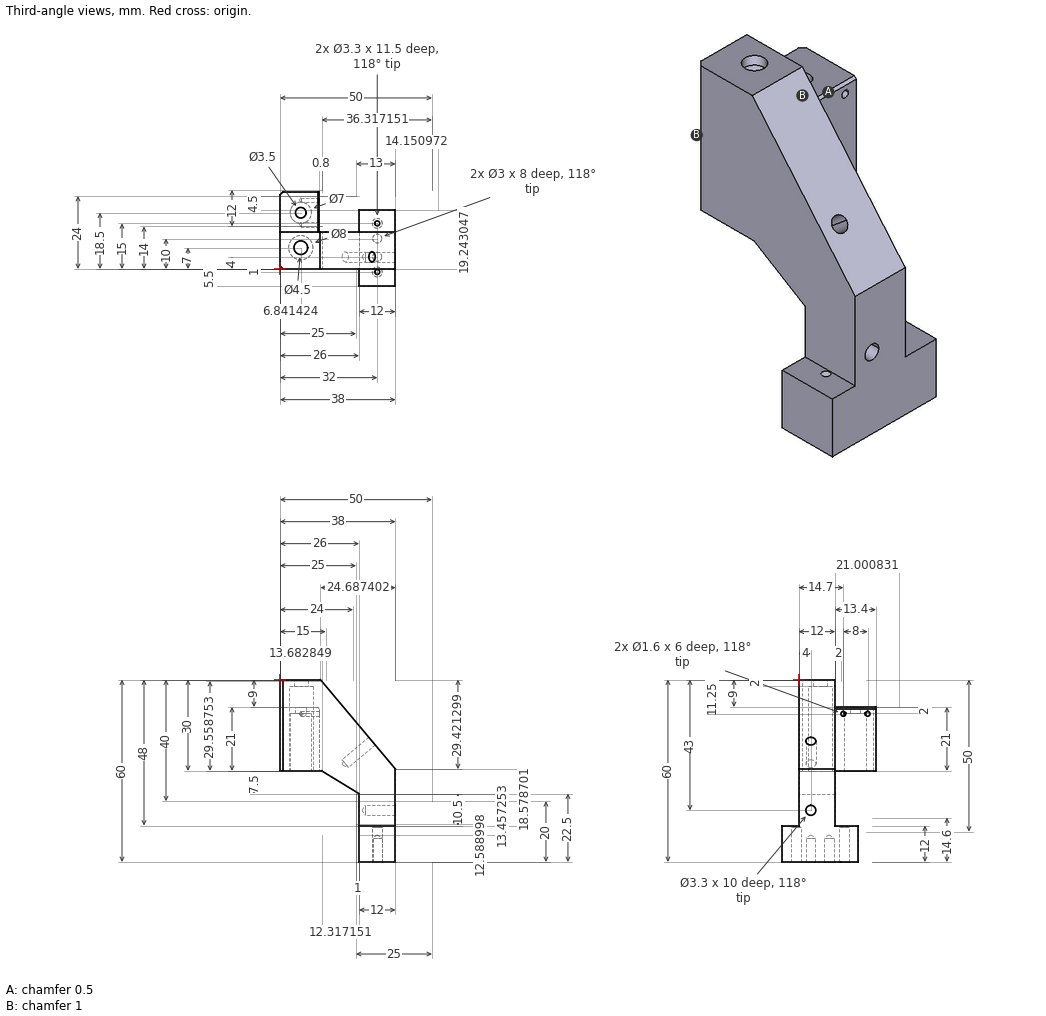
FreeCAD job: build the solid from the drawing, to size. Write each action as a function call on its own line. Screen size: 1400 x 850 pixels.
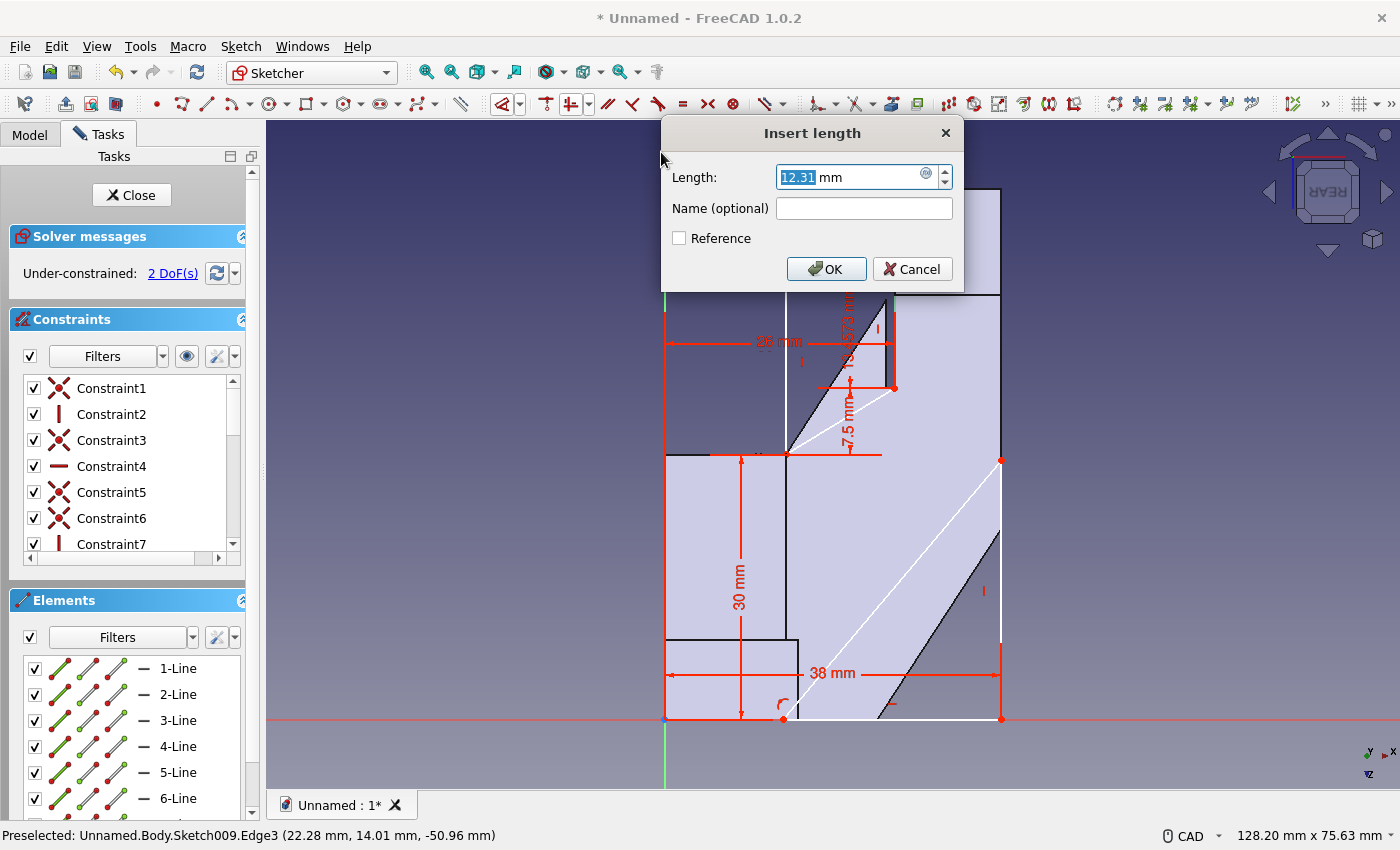
text(12.317151)
key(Return)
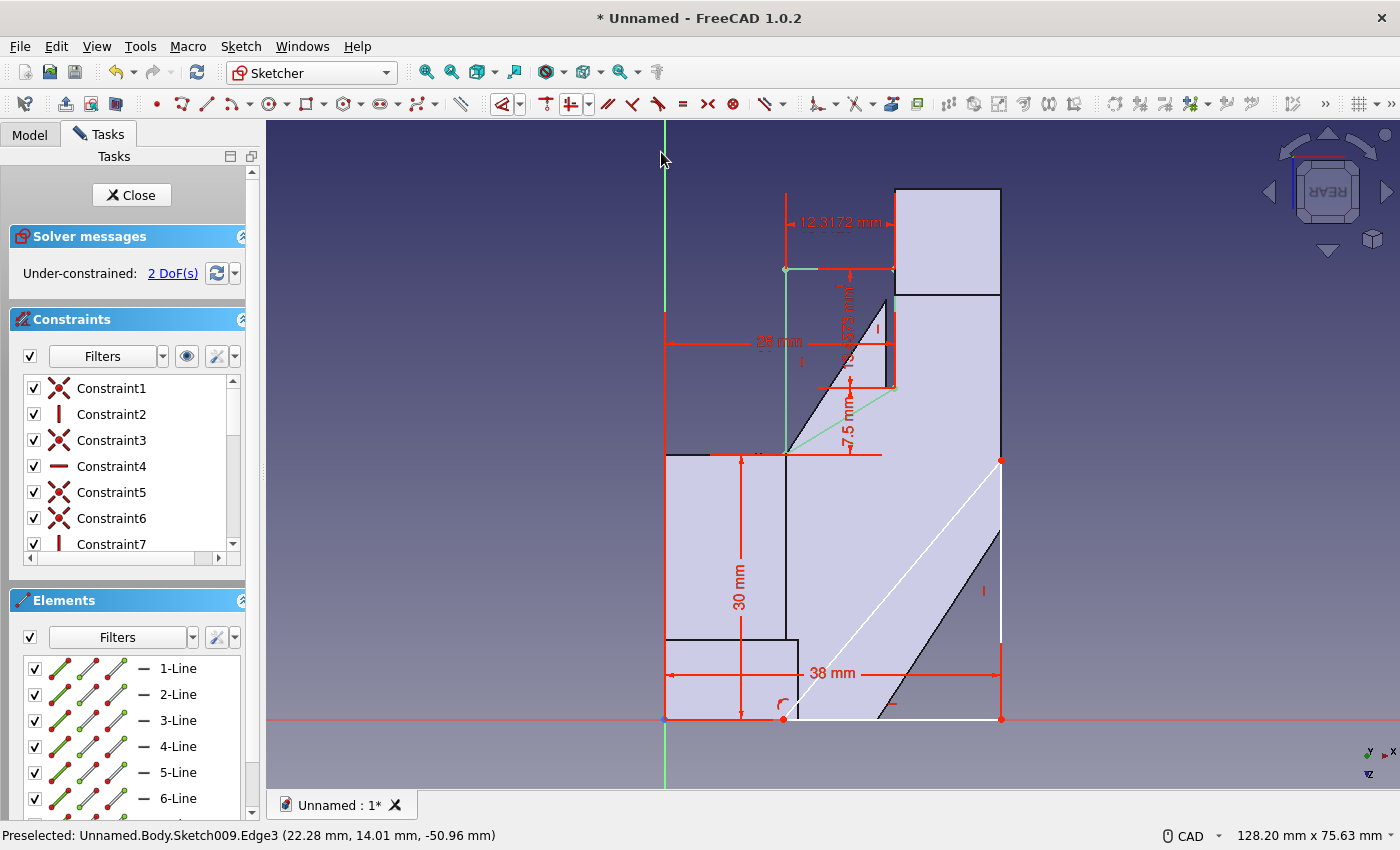
click(848, 720)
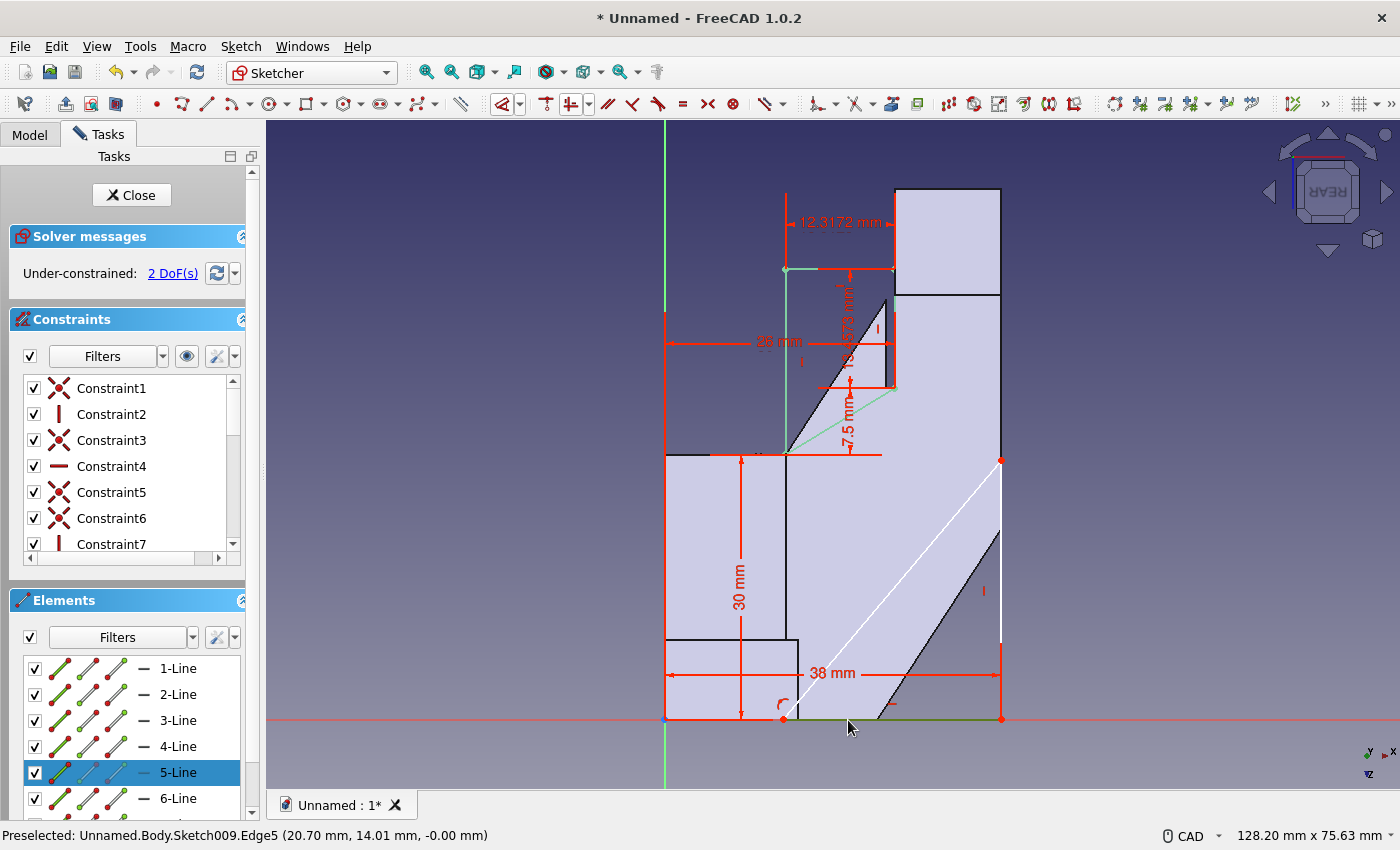
key(l)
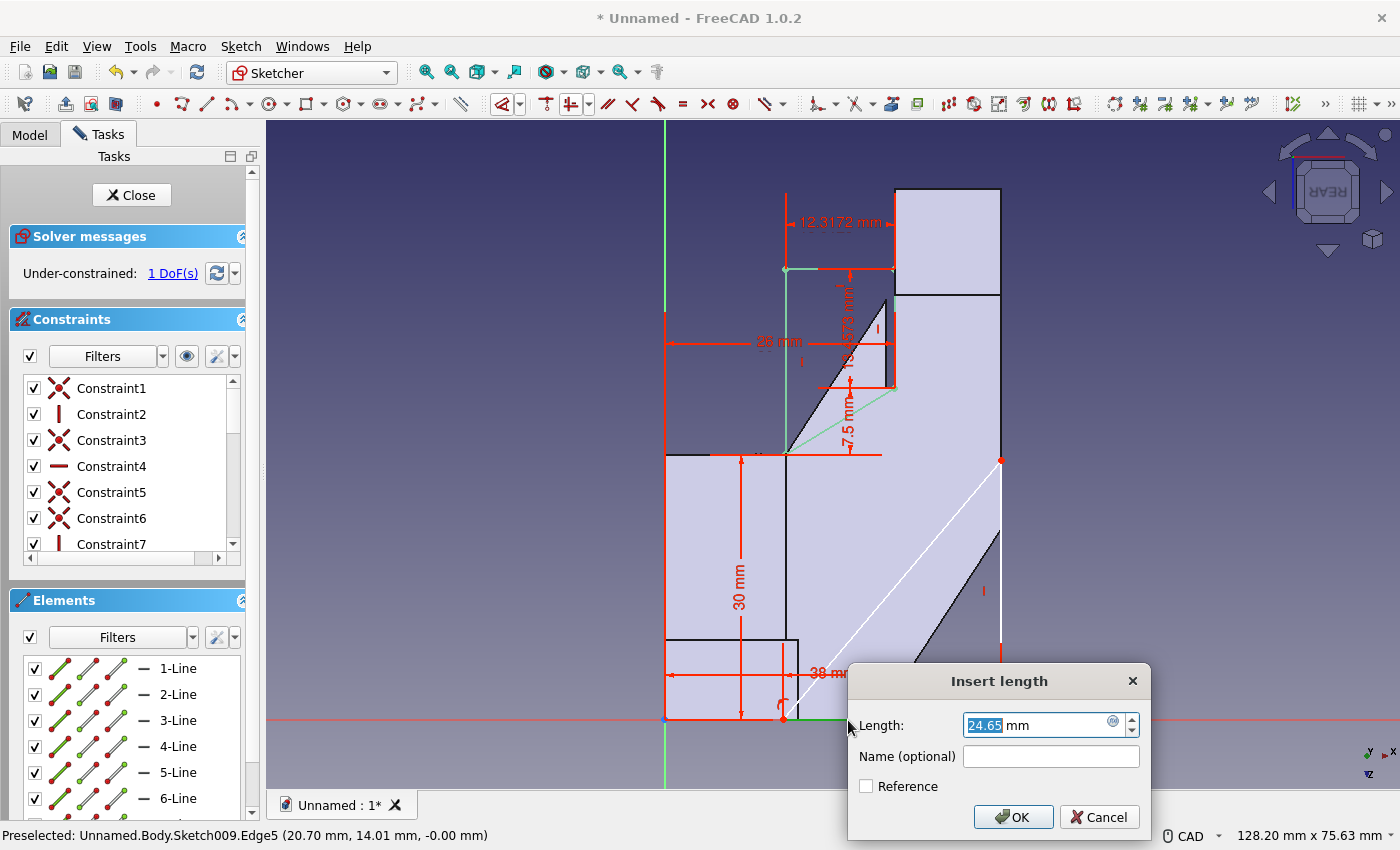
text(24.687402)
key(Return)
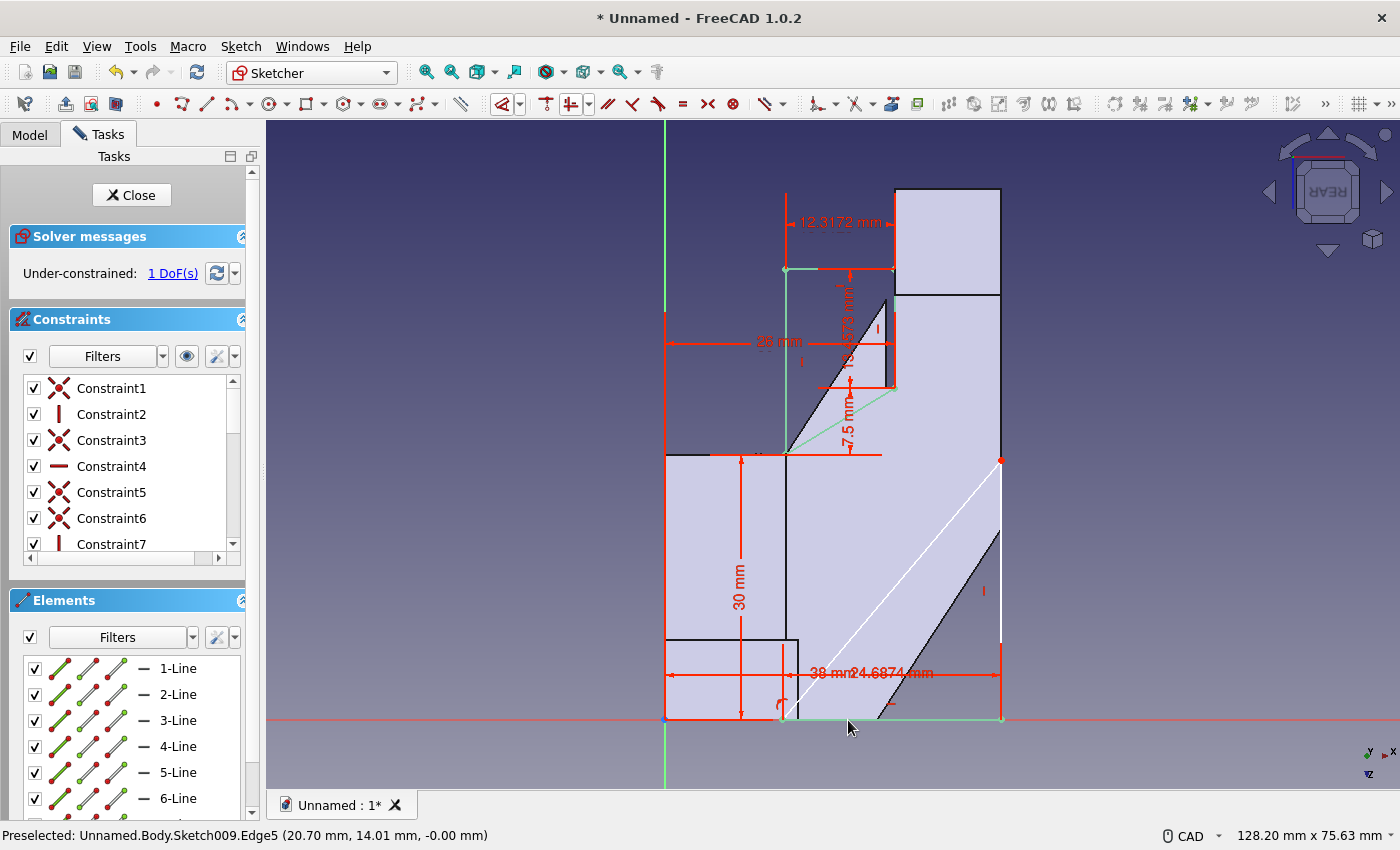
click(1001, 642)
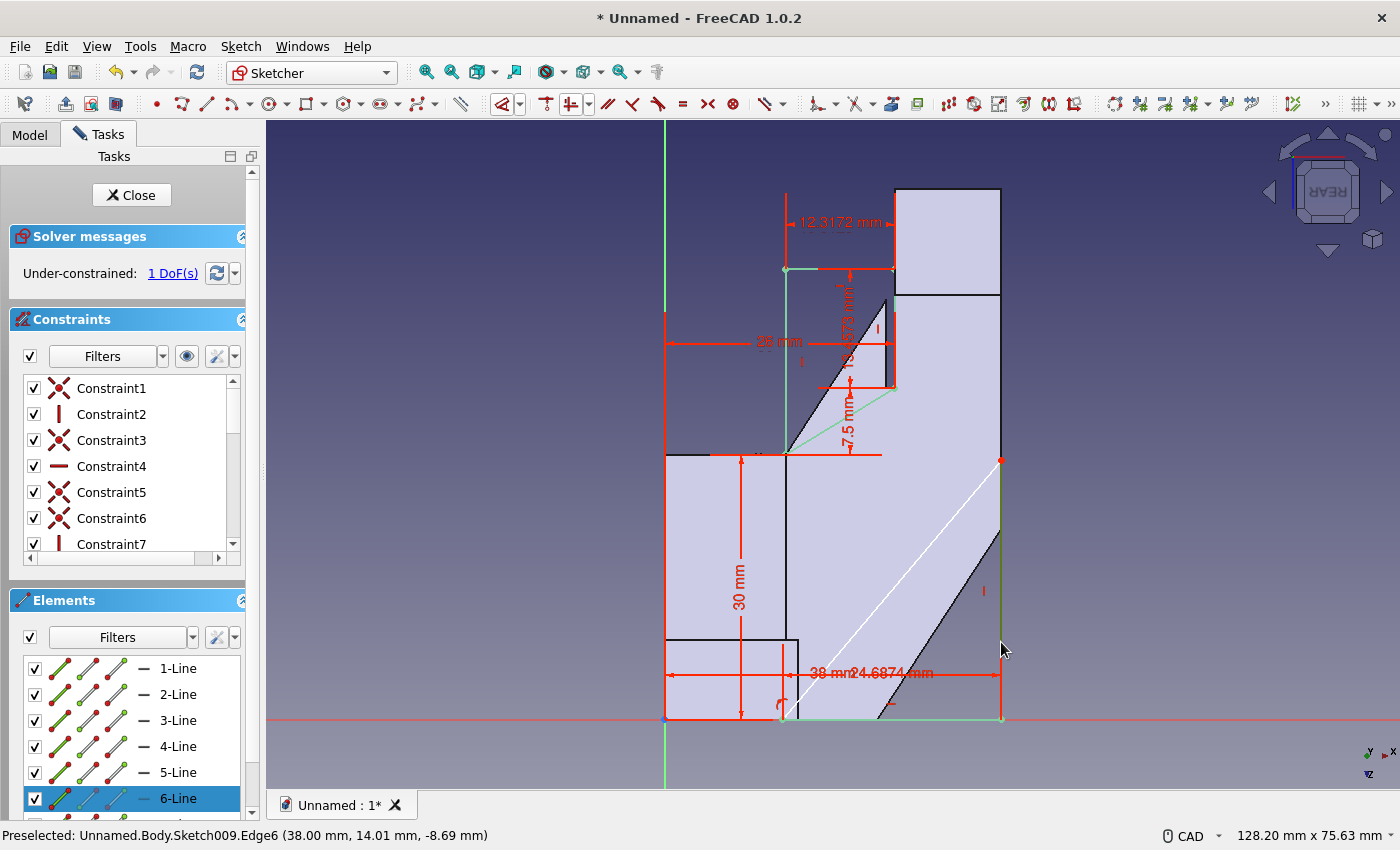
click(520, 104)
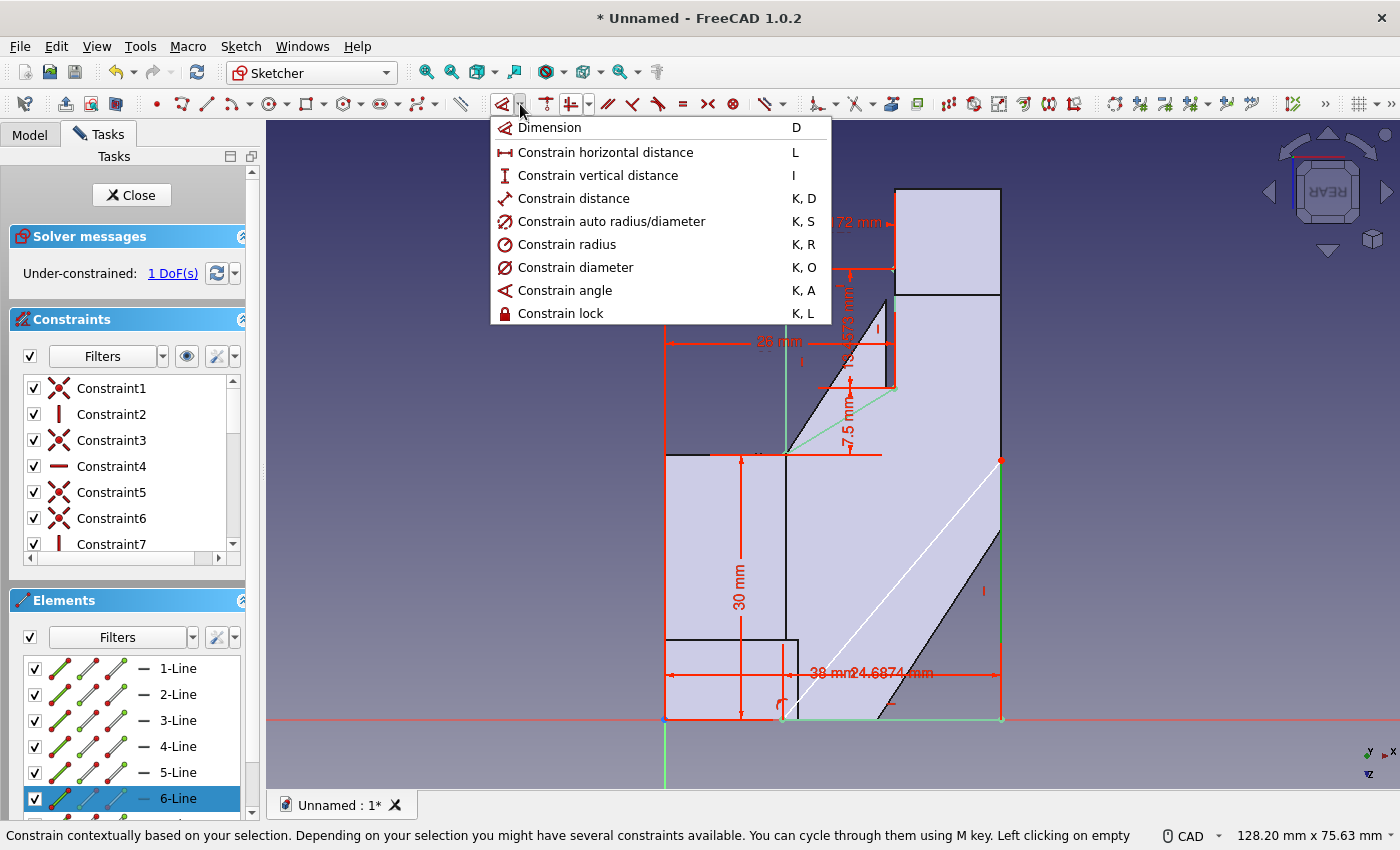
click(661, 176)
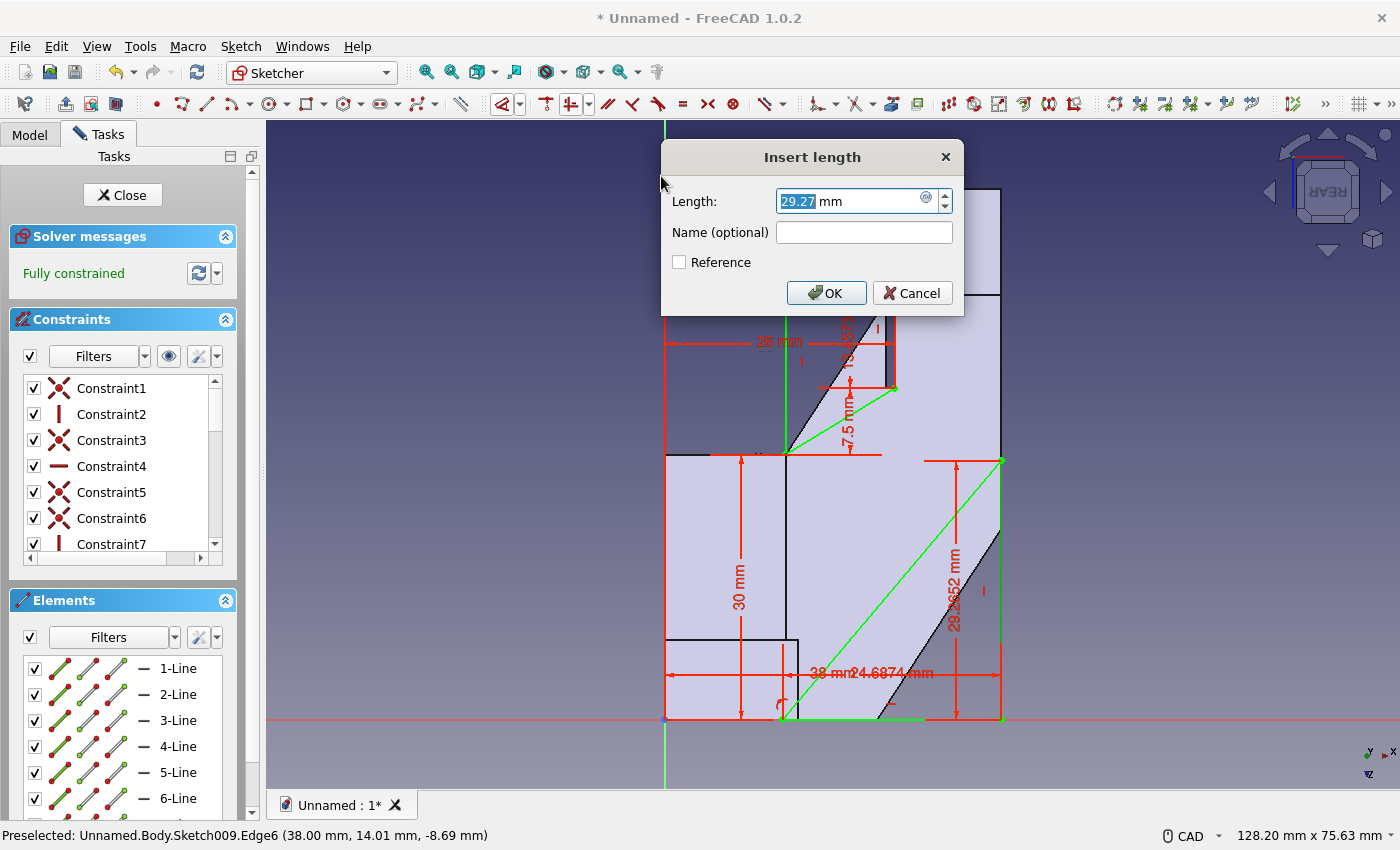
text(29.421299)
key(Return)